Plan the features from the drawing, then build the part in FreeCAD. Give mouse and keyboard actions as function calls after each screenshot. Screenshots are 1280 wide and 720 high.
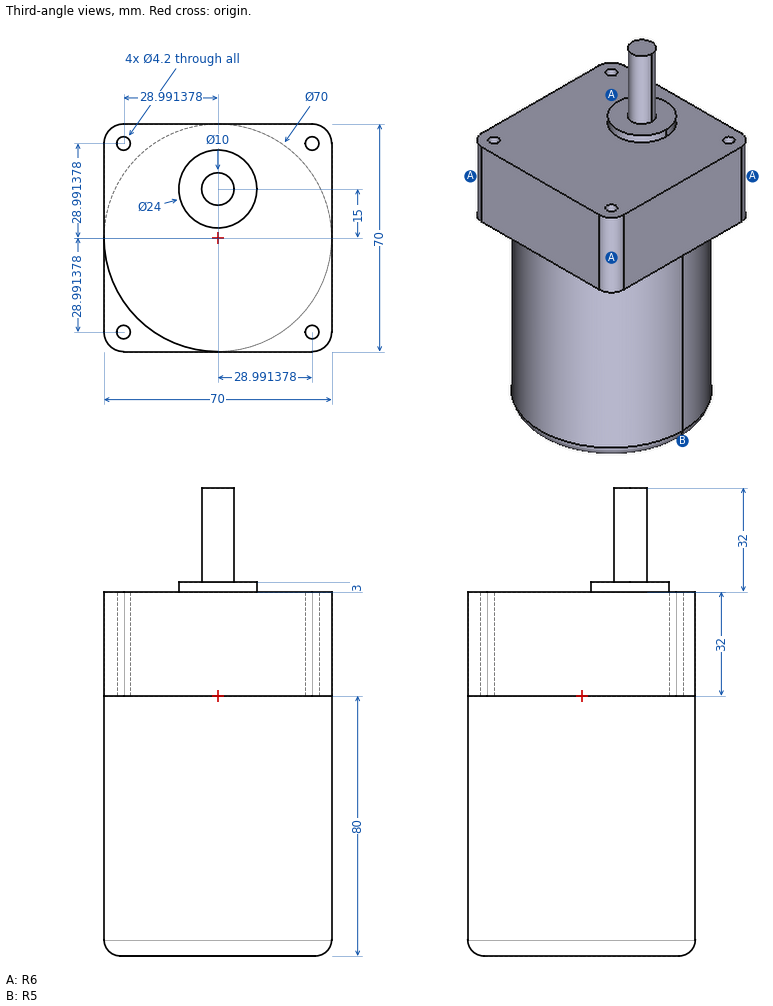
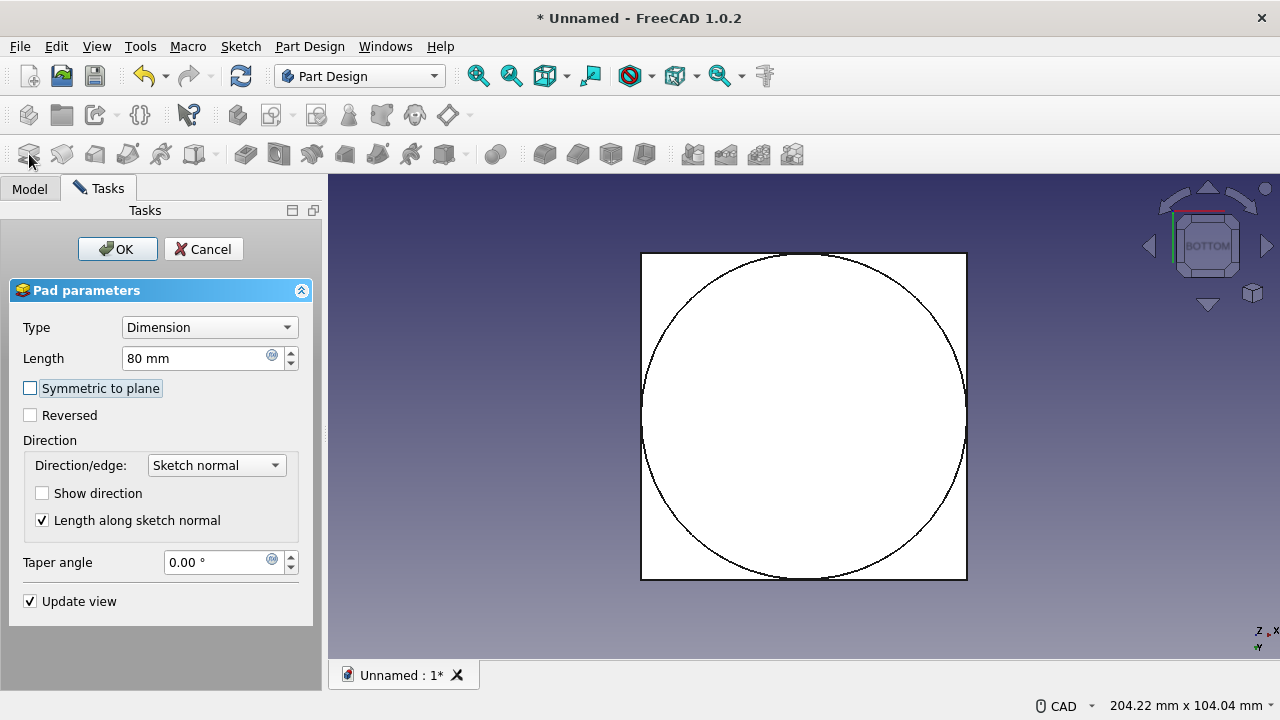
click(118, 249)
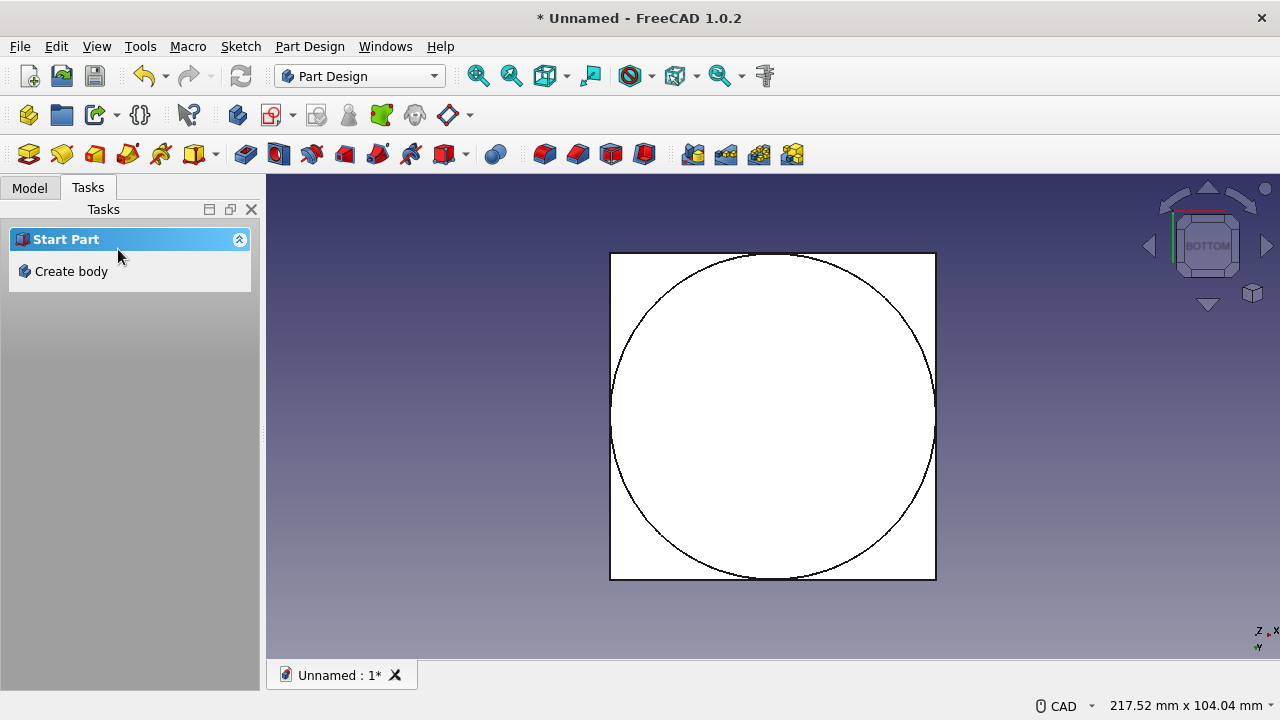
key(0)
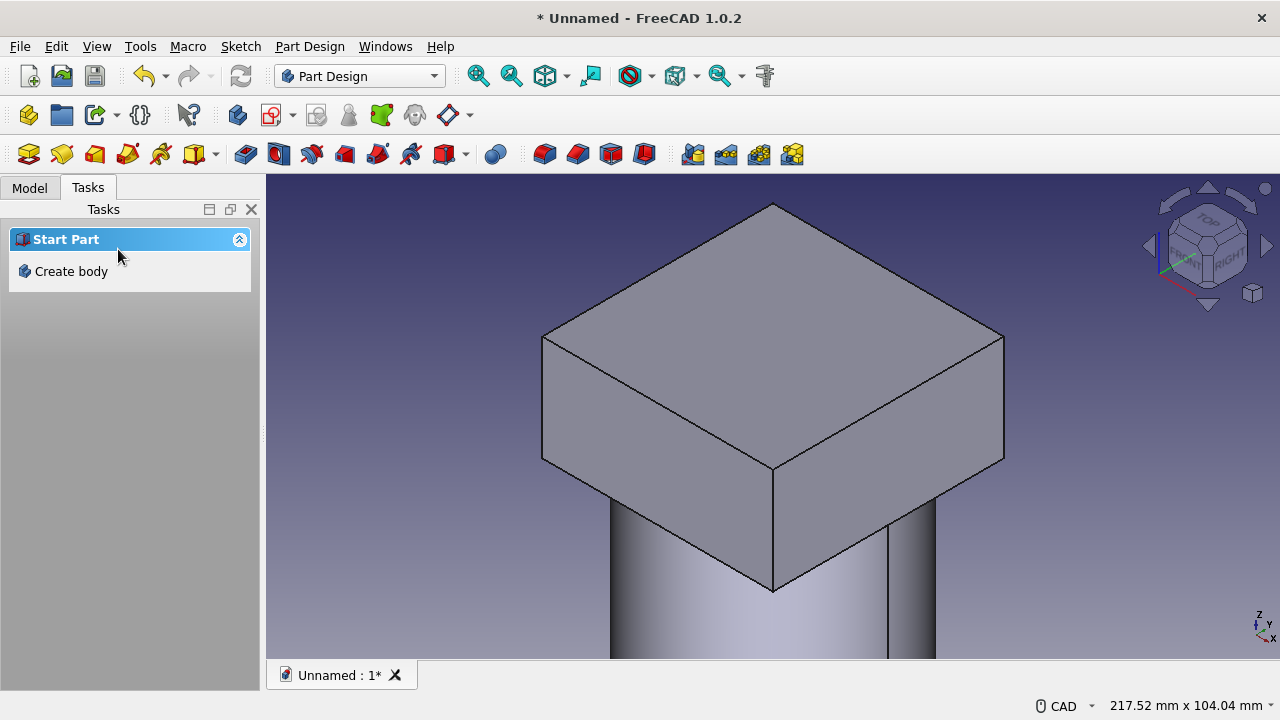
click(479, 76)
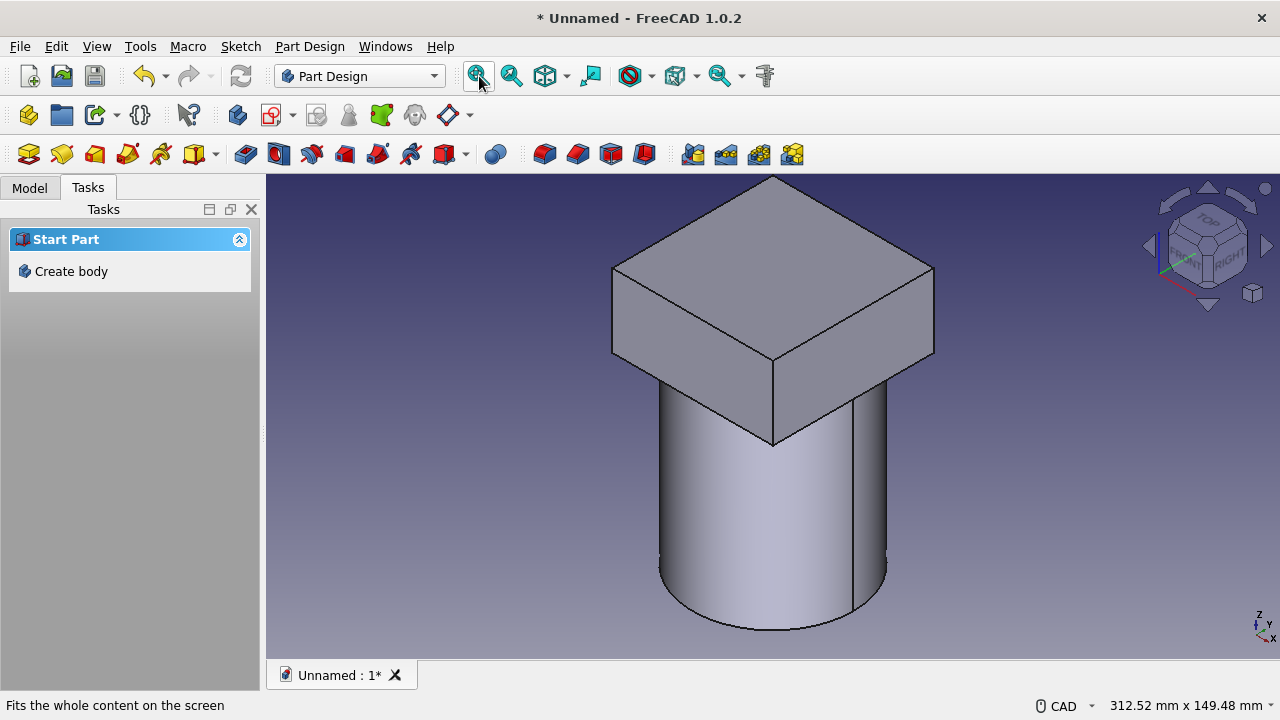
click(773, 402)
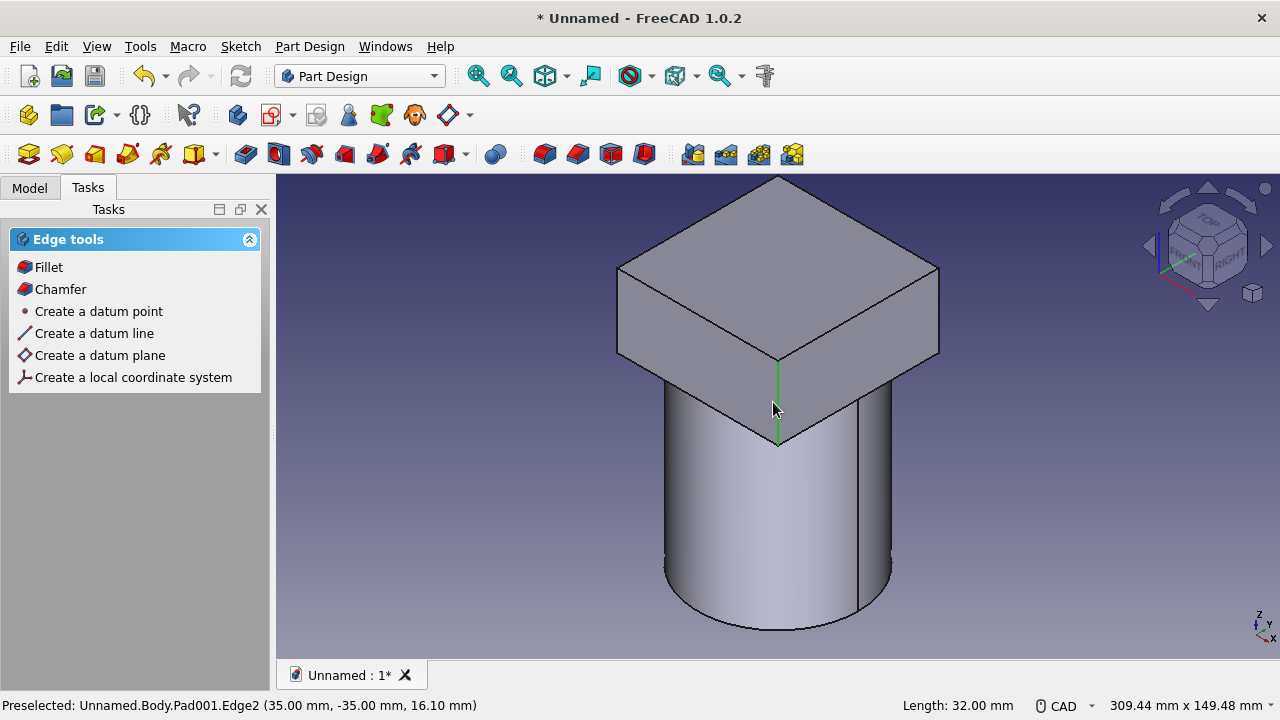
key(2)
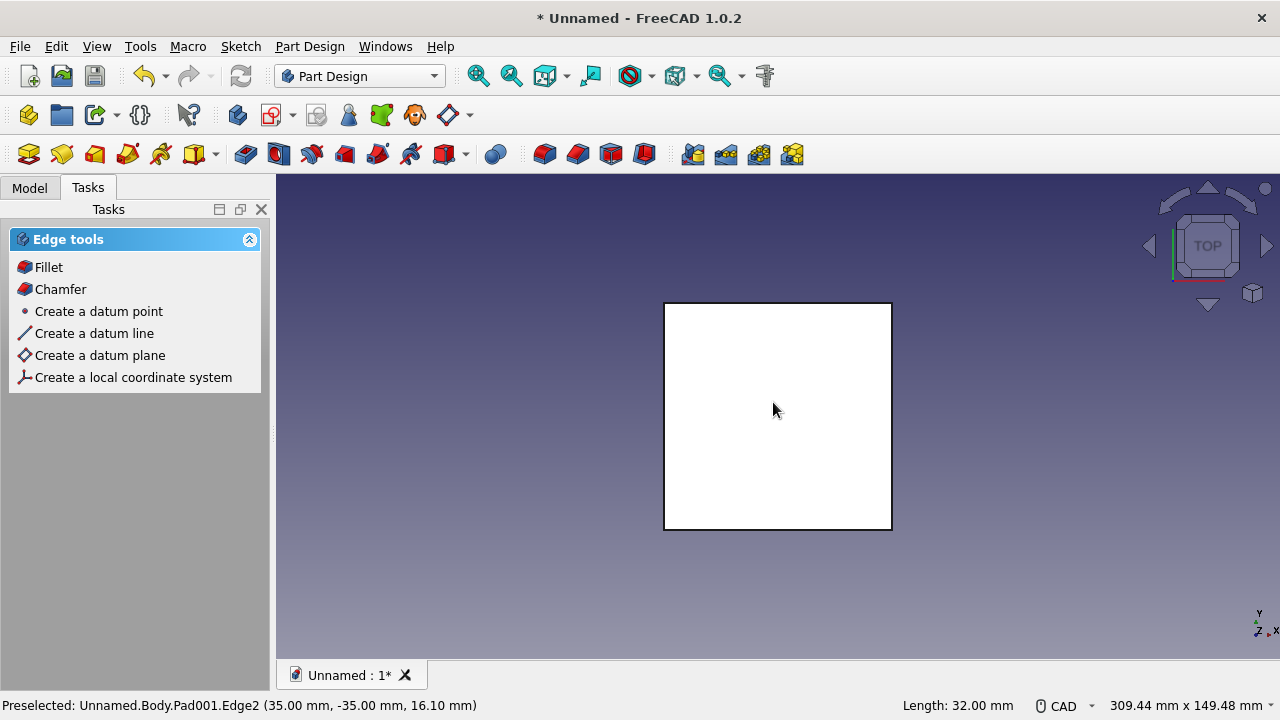
key(1)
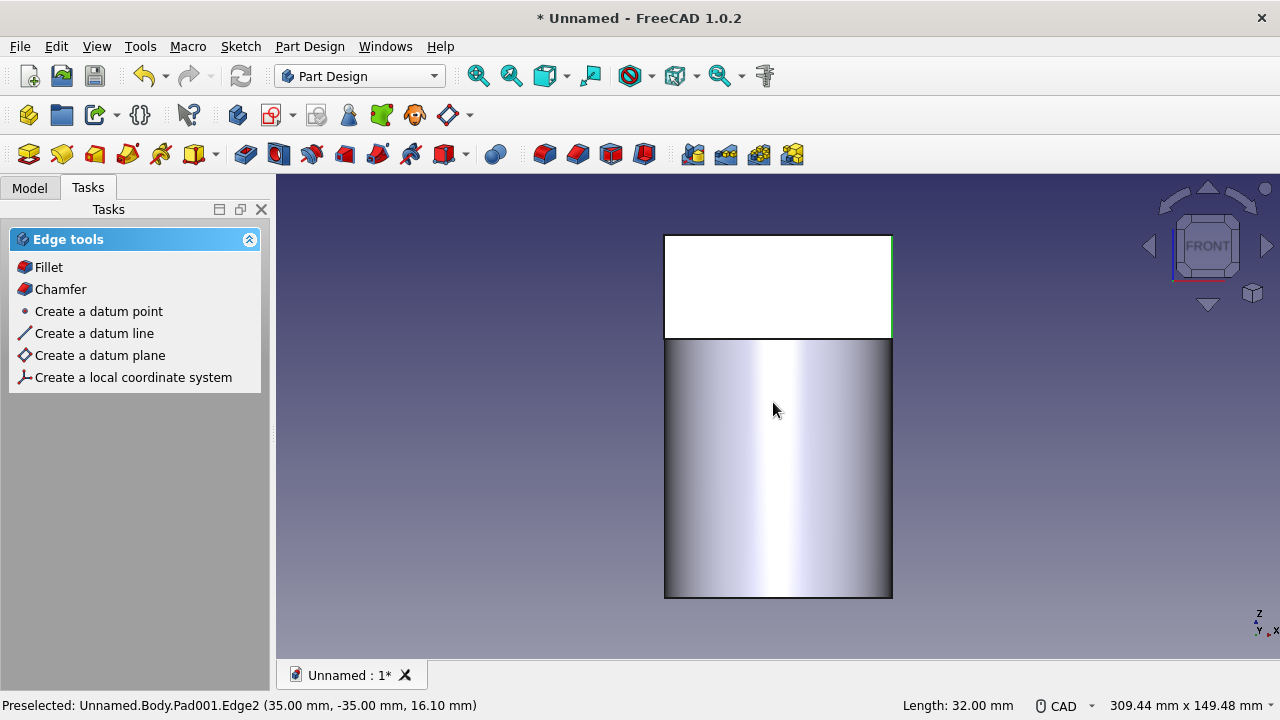
click(664, 286, ctrl)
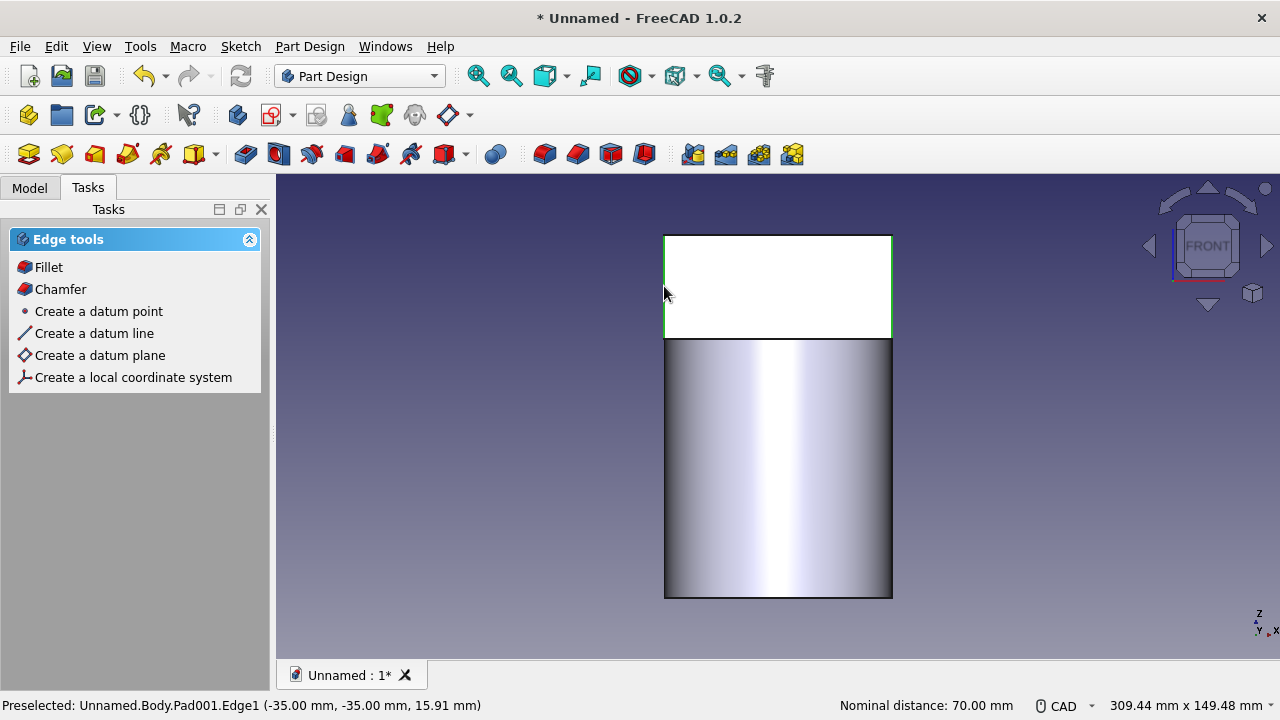
key(3)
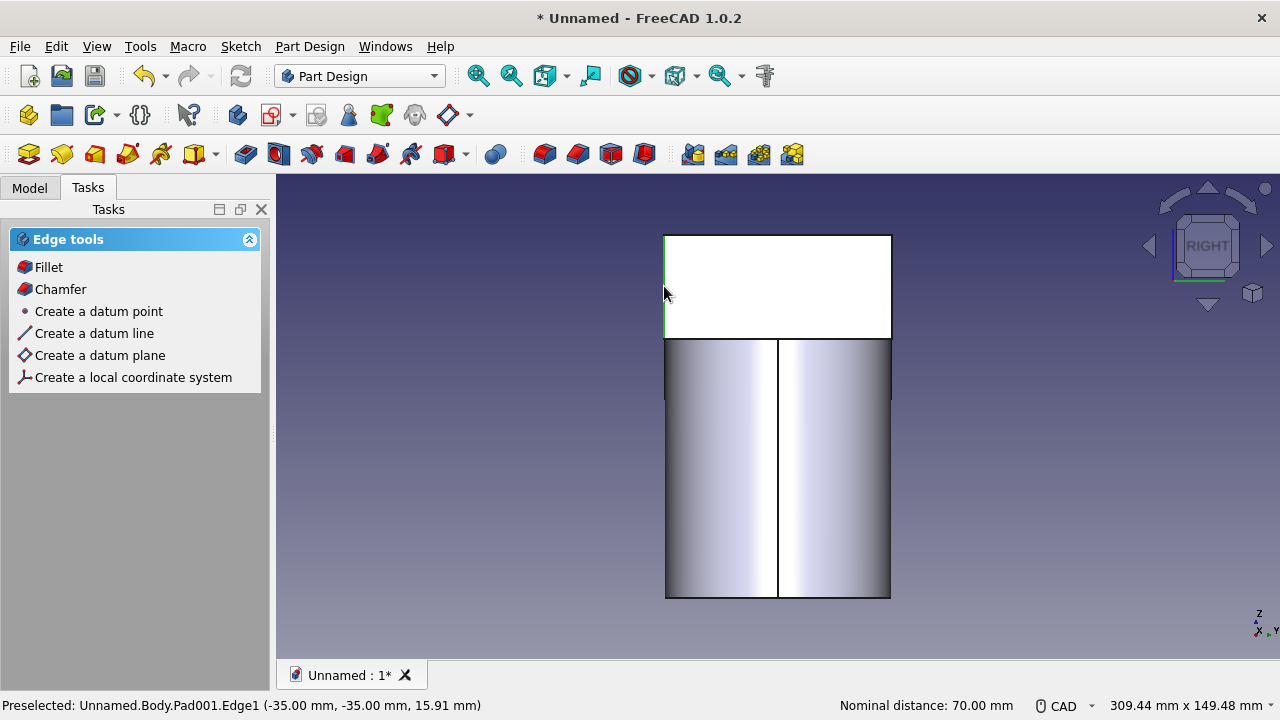
click(892, 286, ctrl)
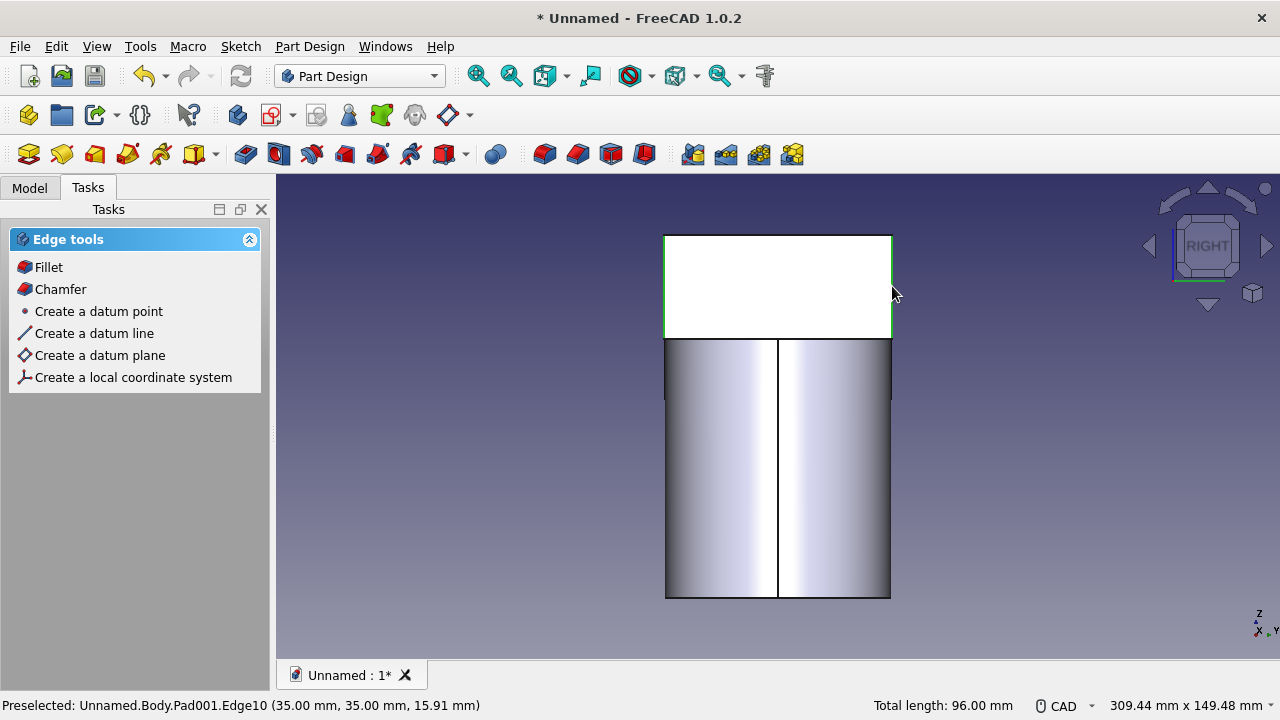
key(5)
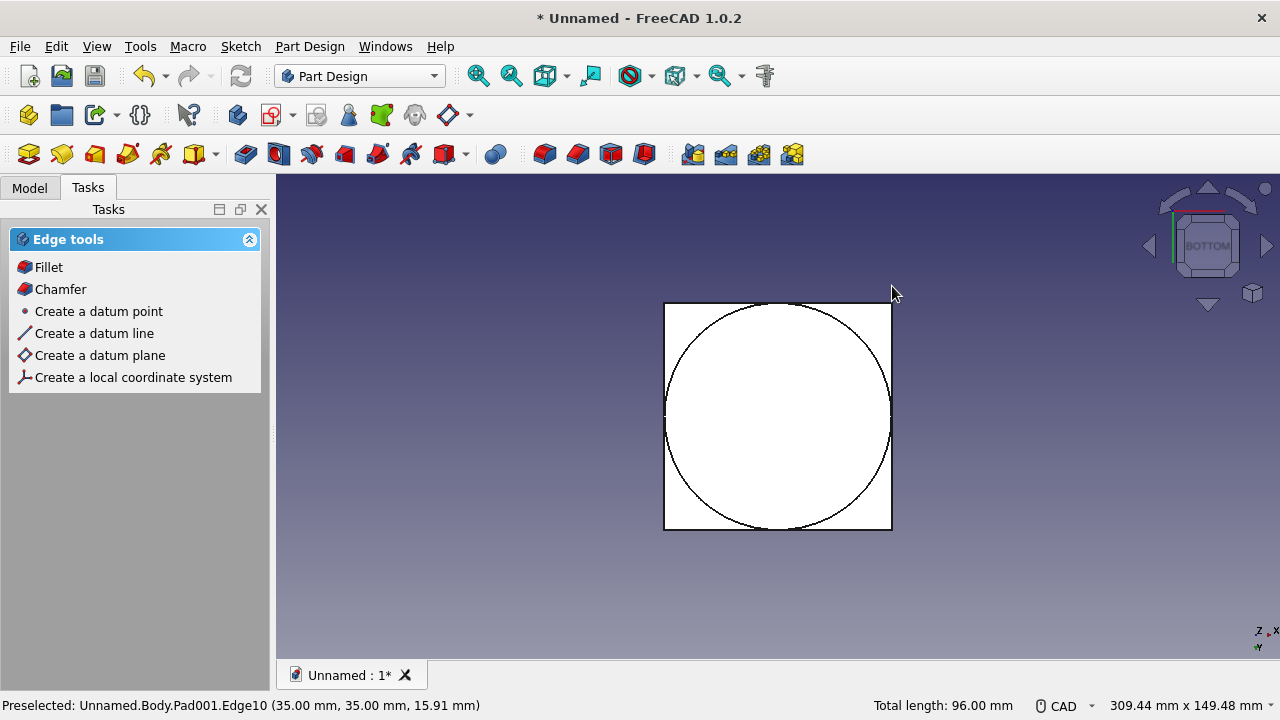
key(4)